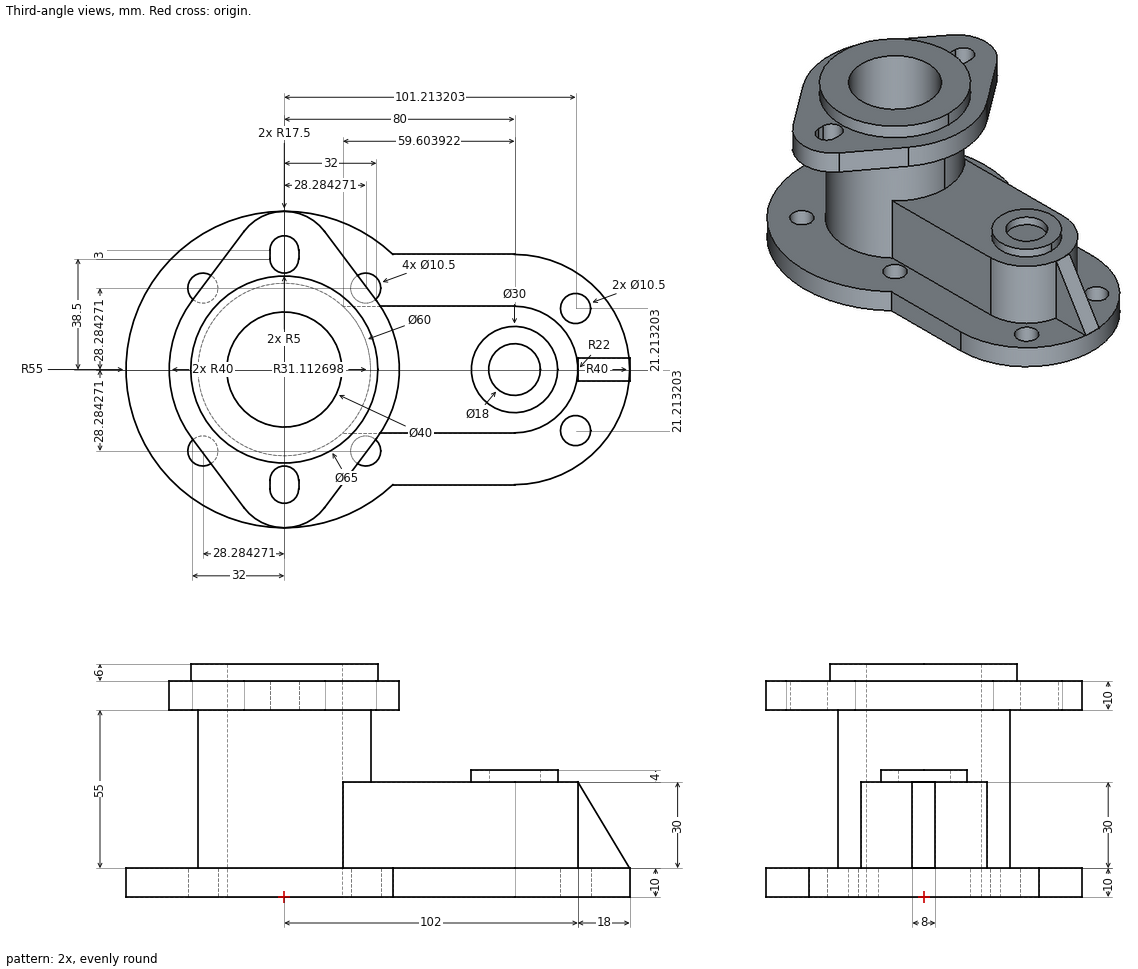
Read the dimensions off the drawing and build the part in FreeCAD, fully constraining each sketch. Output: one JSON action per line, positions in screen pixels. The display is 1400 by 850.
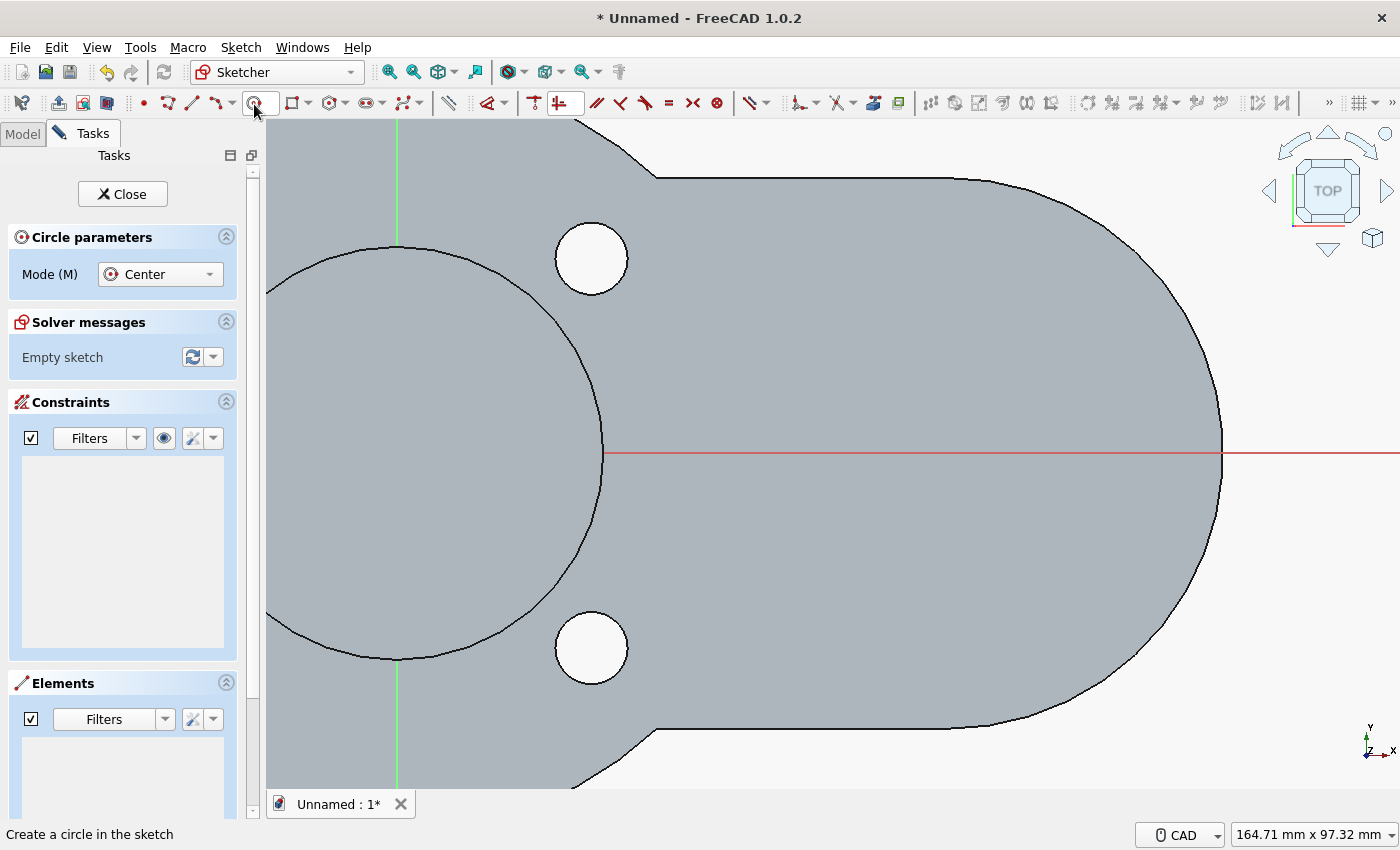
{"action": "left_click", "coordinate": [1094, 307]}
{"action": "mouse_move", "coordinate": [1119, 282]}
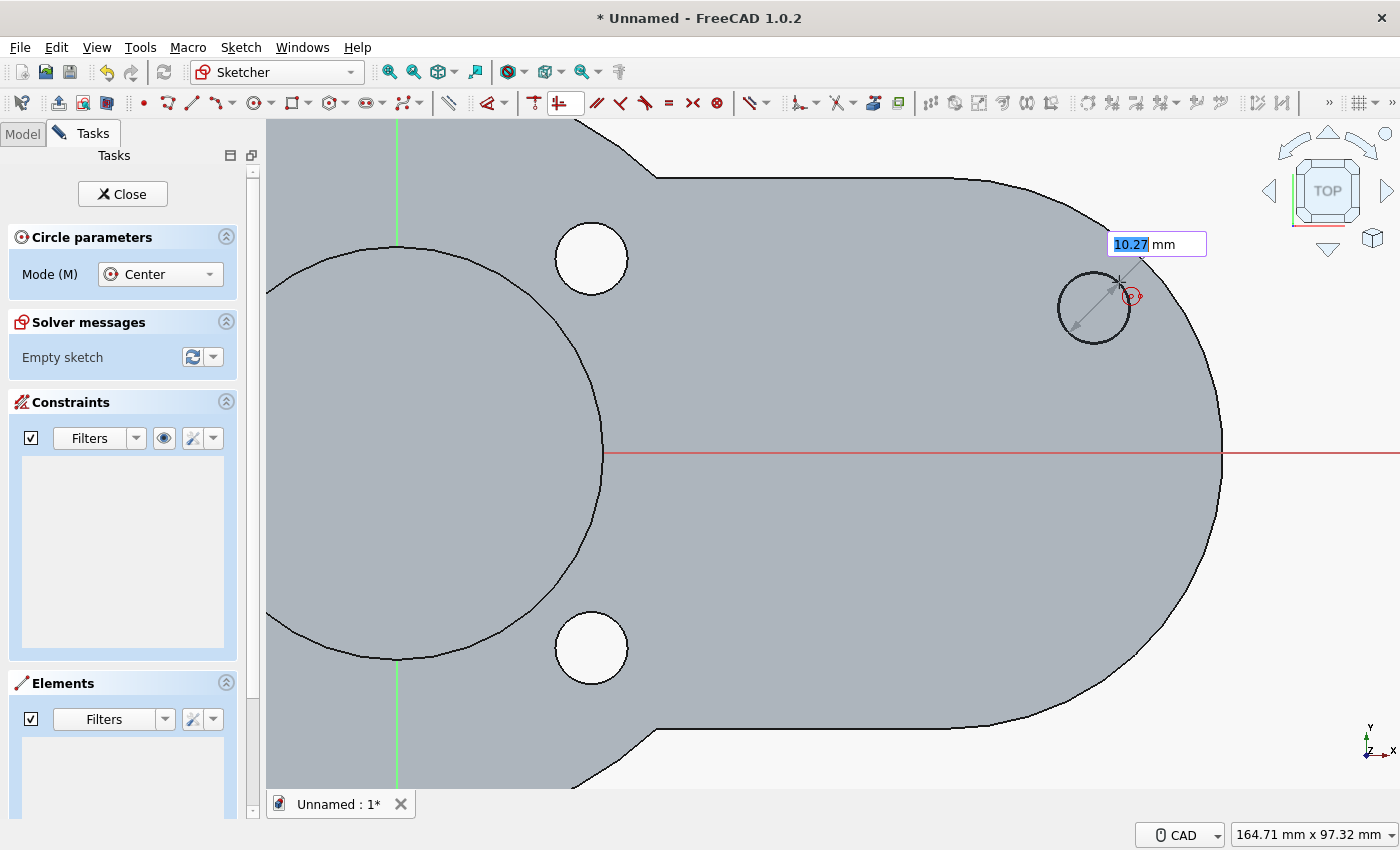
{"action": "type", "text": "10.5"}
{"action": "key", "text": "Return"}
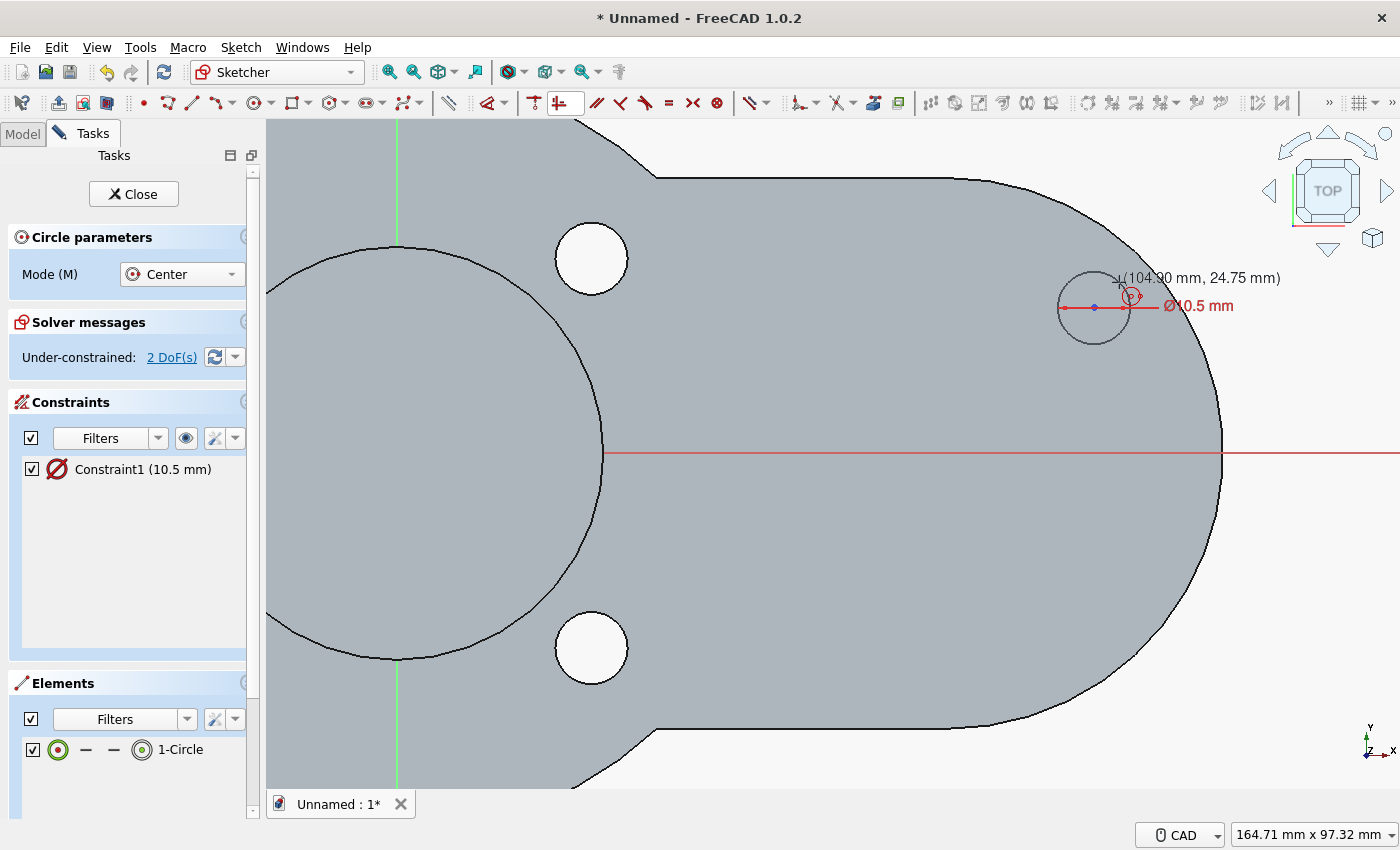
{"action": "left_click", "coordinate": [1094, 599]}
{"action": "mouse_move", "coordinate": [1119, 574]}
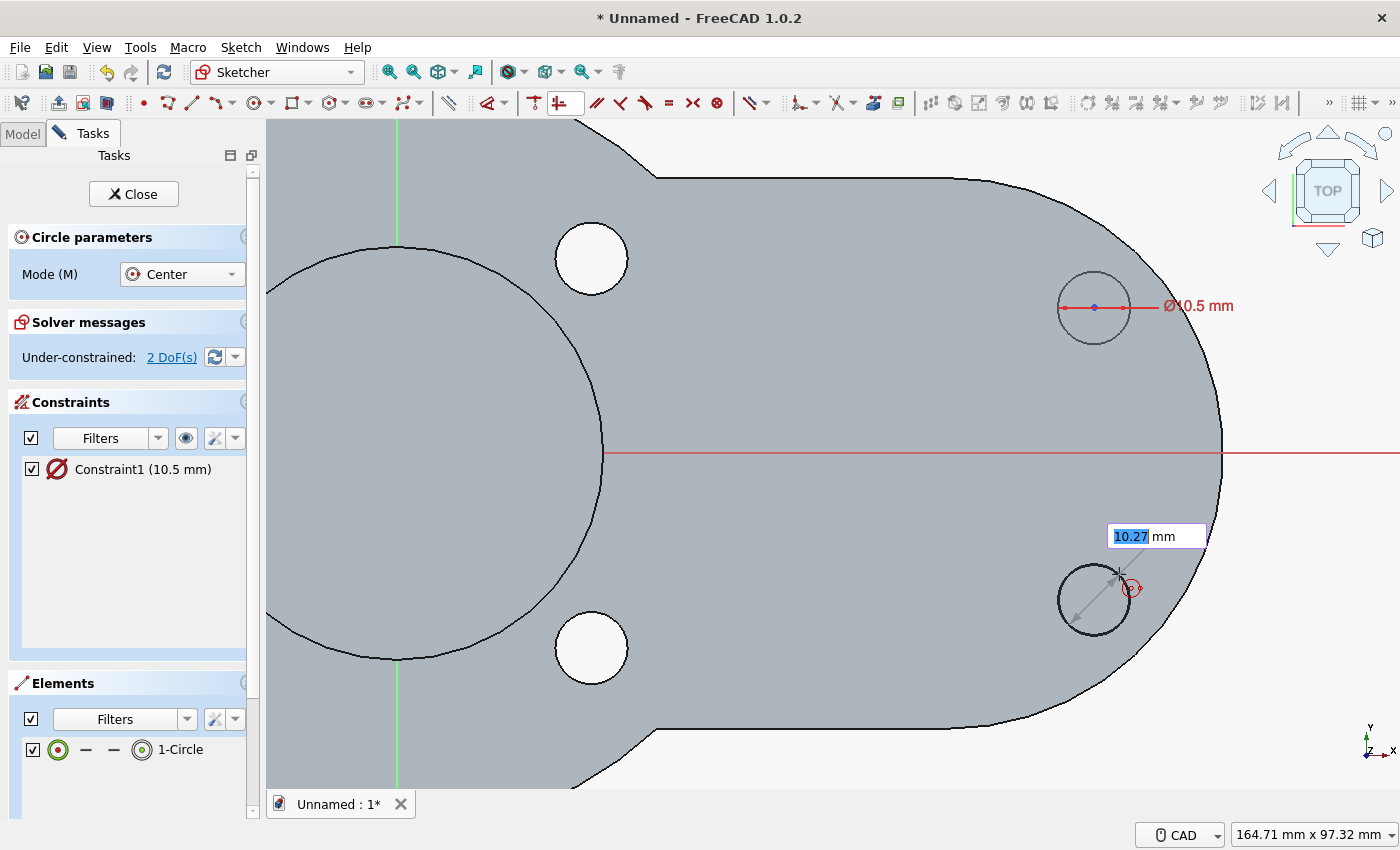
{"action": "type", "text": "10.5"}
{"action": "key", "text": "Return"}
{"action": "key", "text": "Escape"}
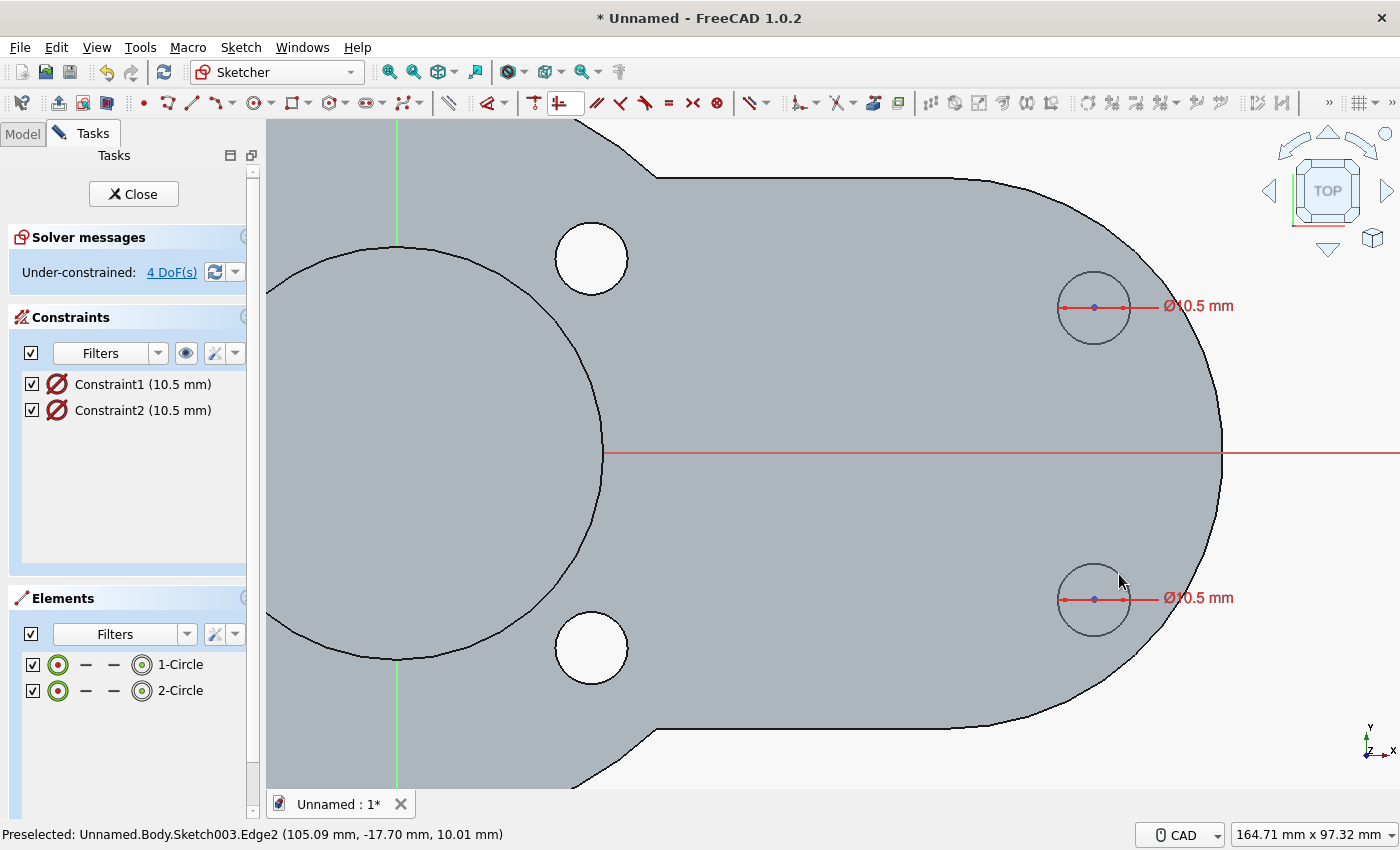
{"action": "left_click", "coordinate": [1094, 308]}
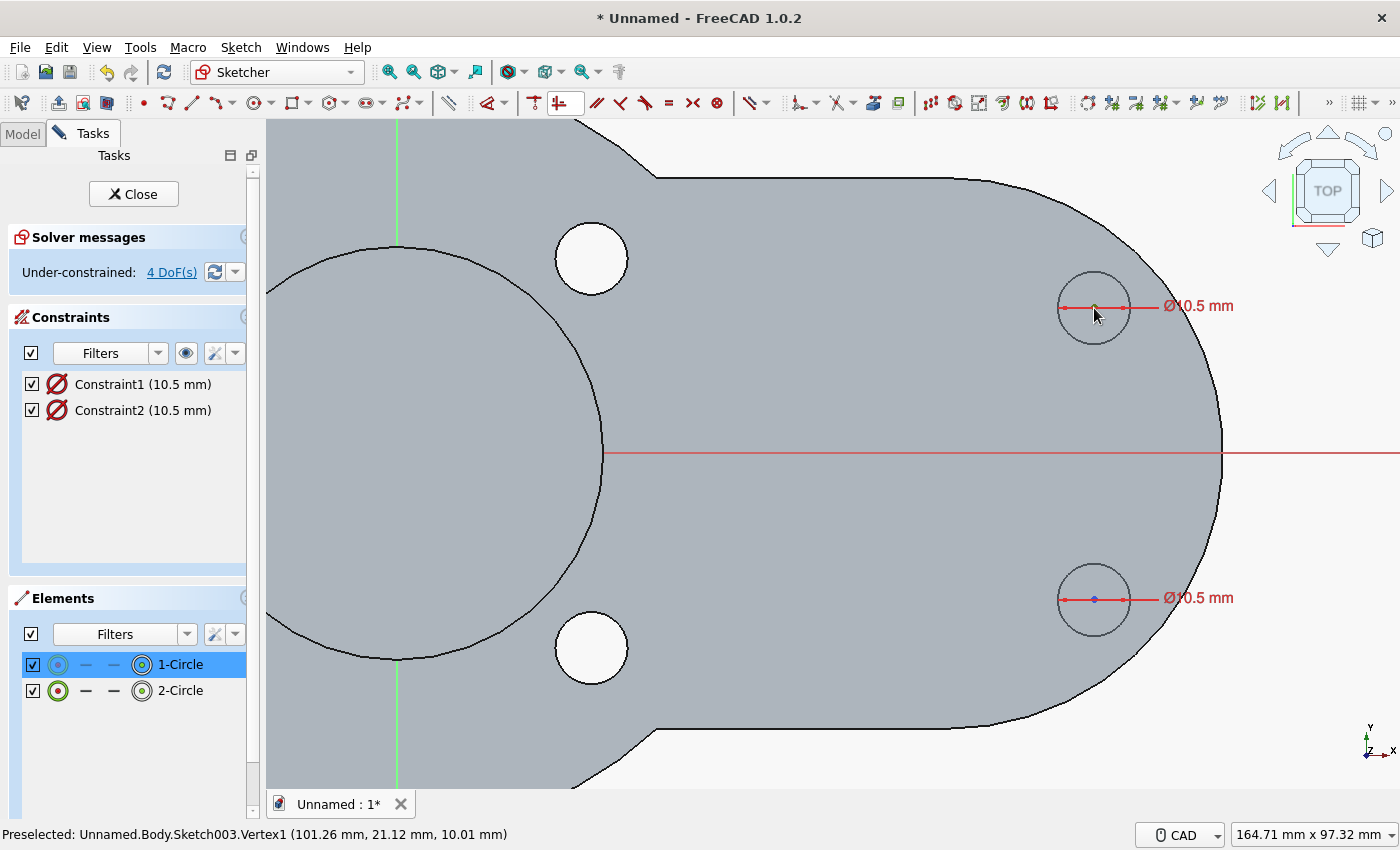
{"action": "left_click", "coordinate": [1094, 600]}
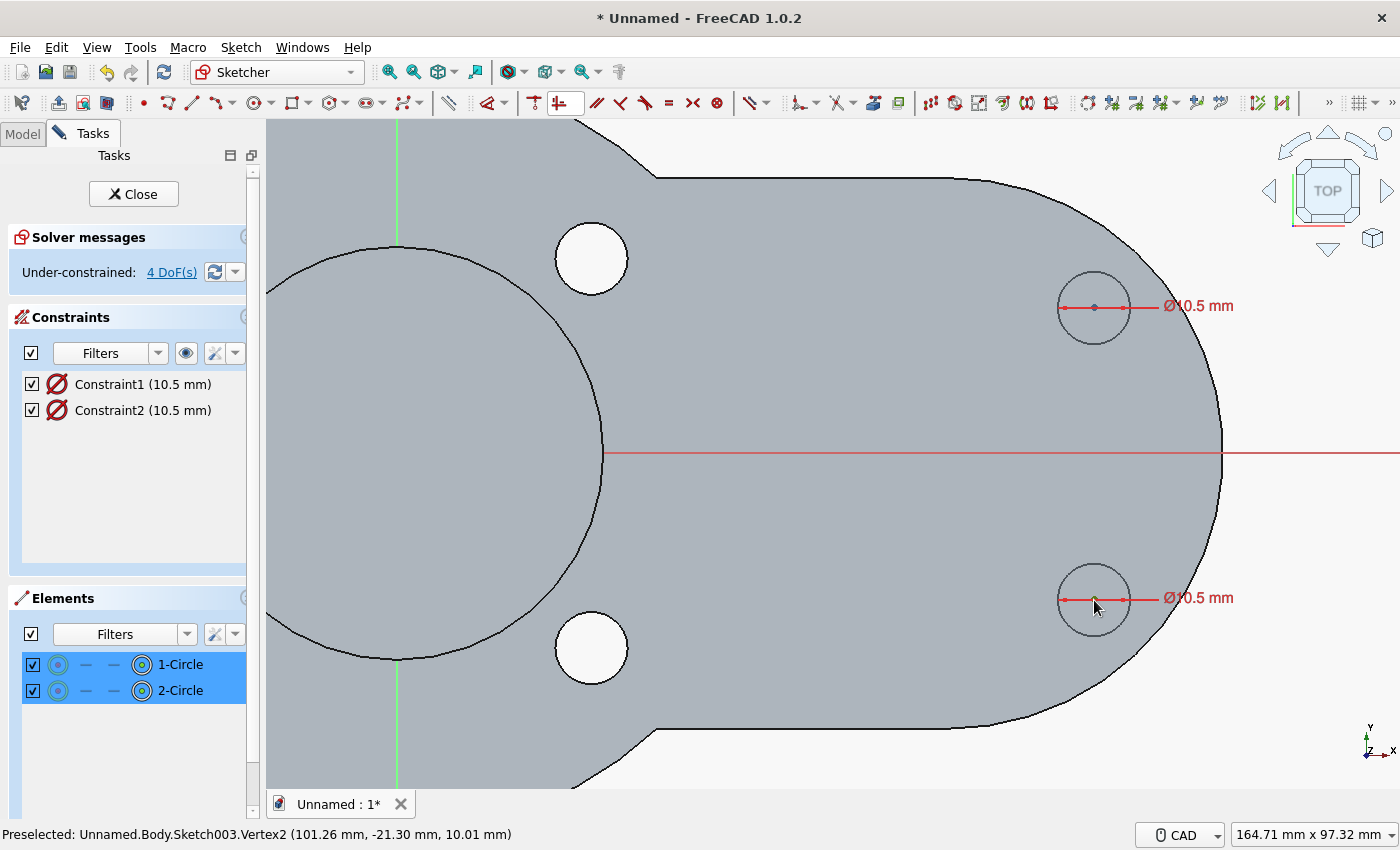
{"action": "left_click", "coordinate": [578, 104]}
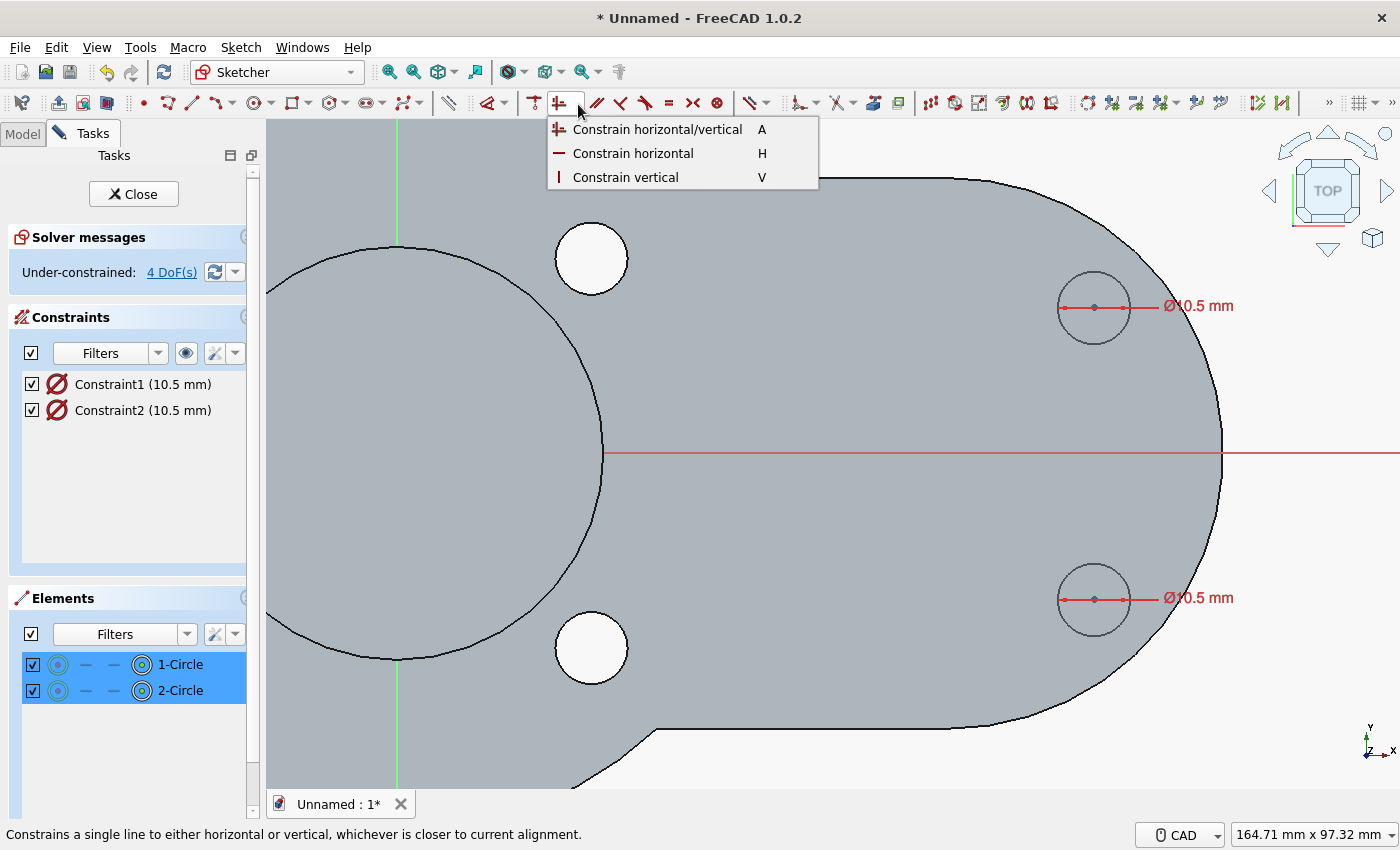
{"action": "left_click", "coordinate": [683, 177]}